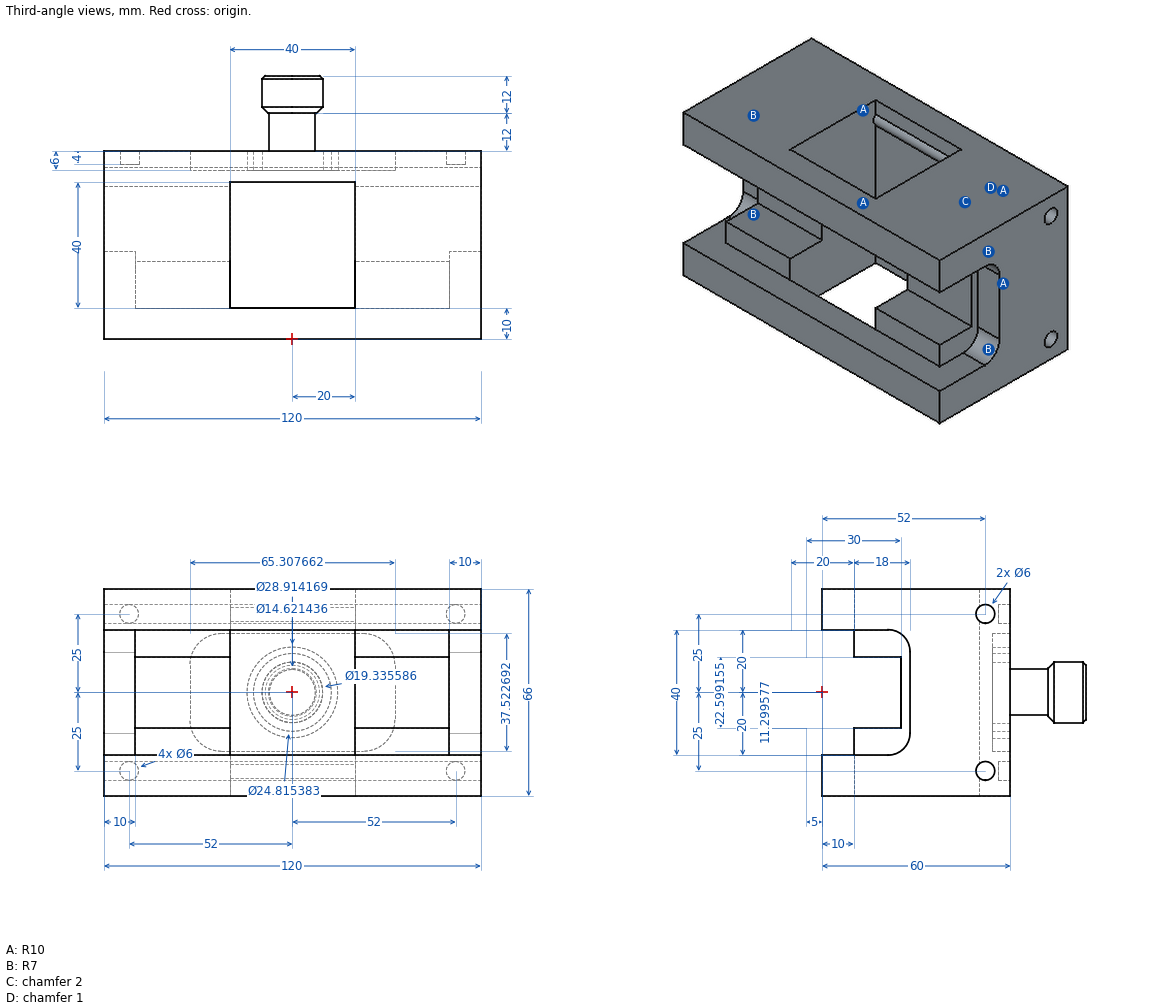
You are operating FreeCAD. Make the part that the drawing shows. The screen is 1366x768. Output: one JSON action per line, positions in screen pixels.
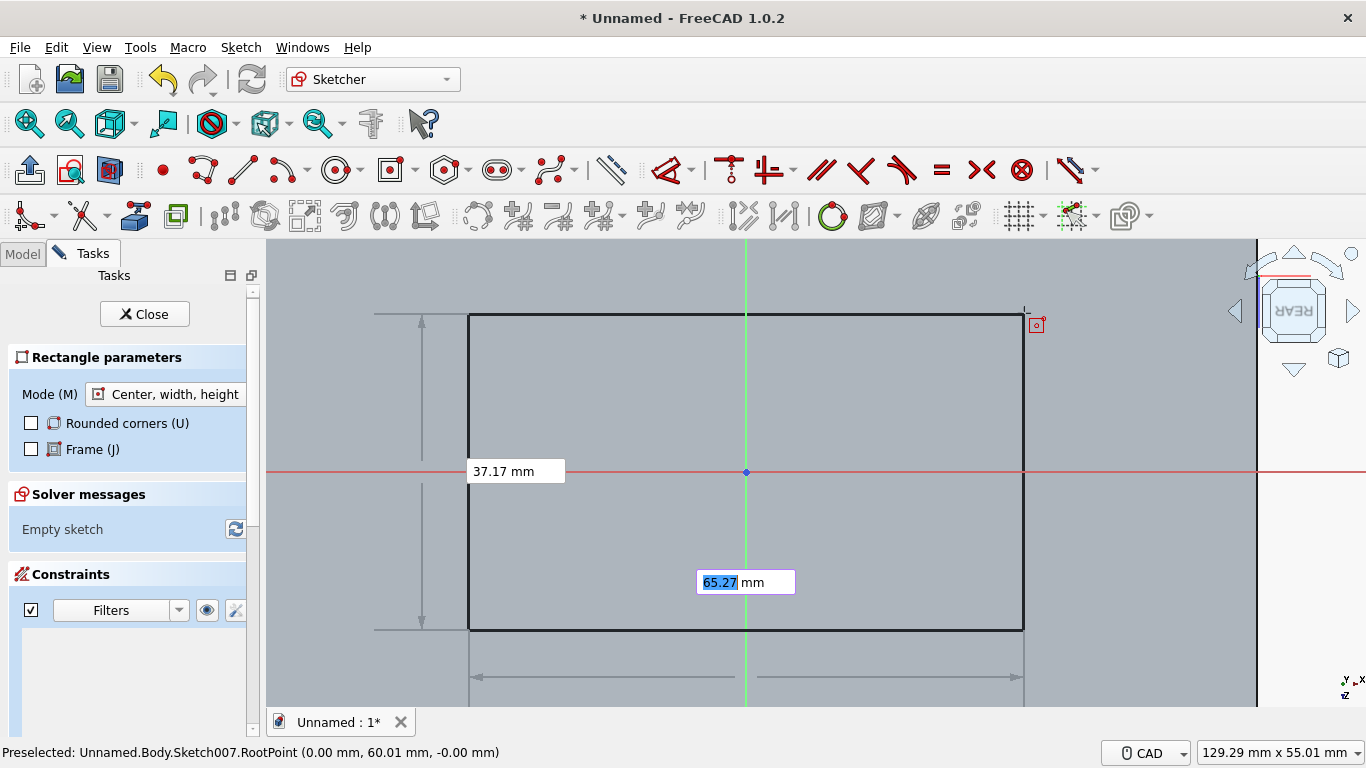
{"action": "type", "text": "65.307662"}
{"action": "key", "text": "Tab"}
{"action": "type", "text": "37.522692"}
{"action": "key", "text": "Return"}
{"action": "key", "text": "Escape"}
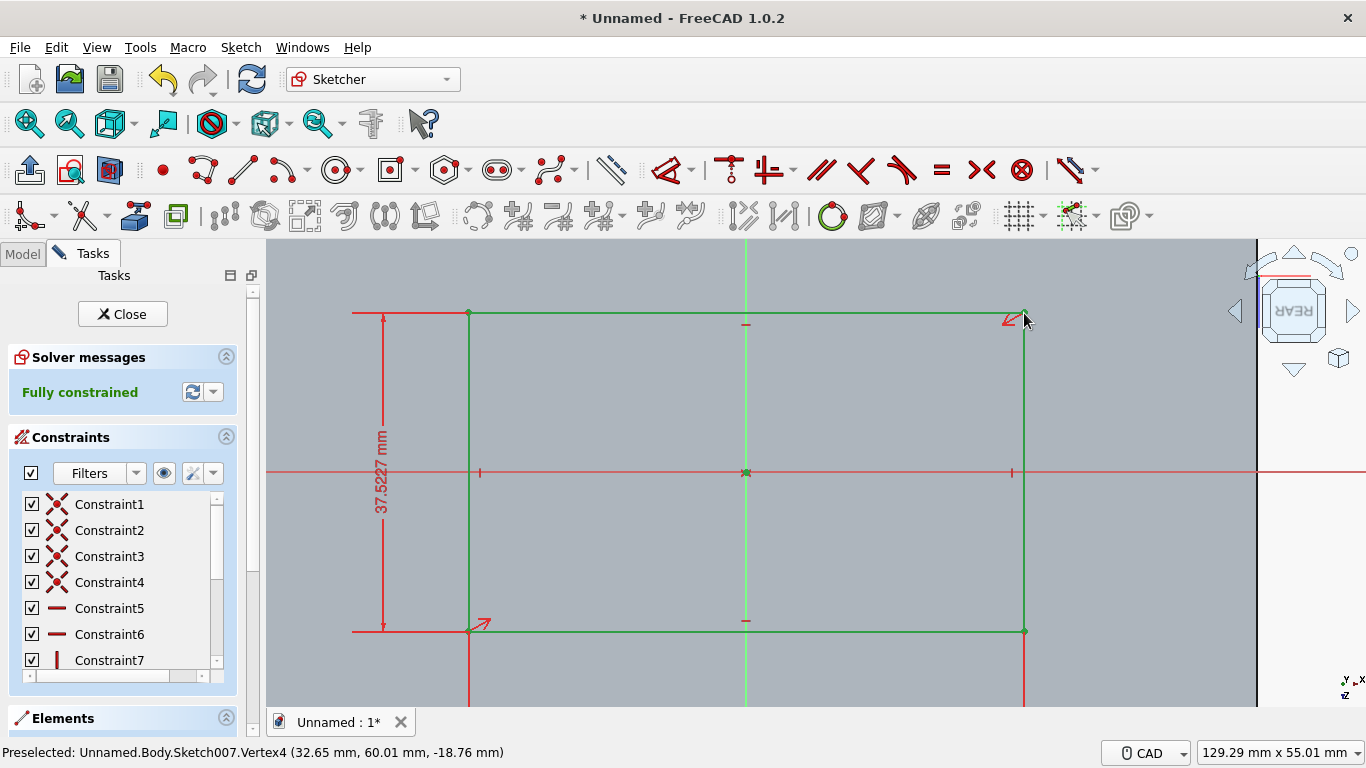
{"action": "left_click", "coordinate": [123, 314]}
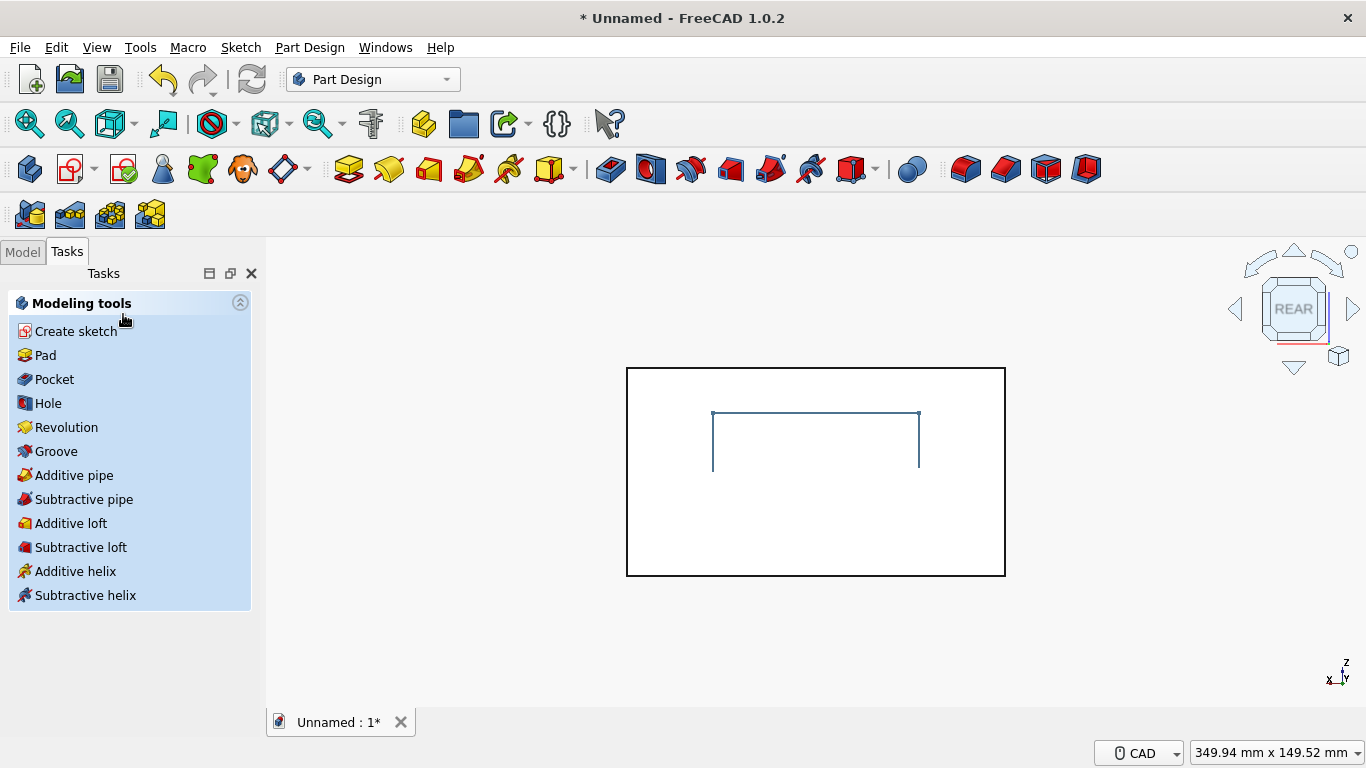
{"action": "left_click", "coordinate": [612, 170]}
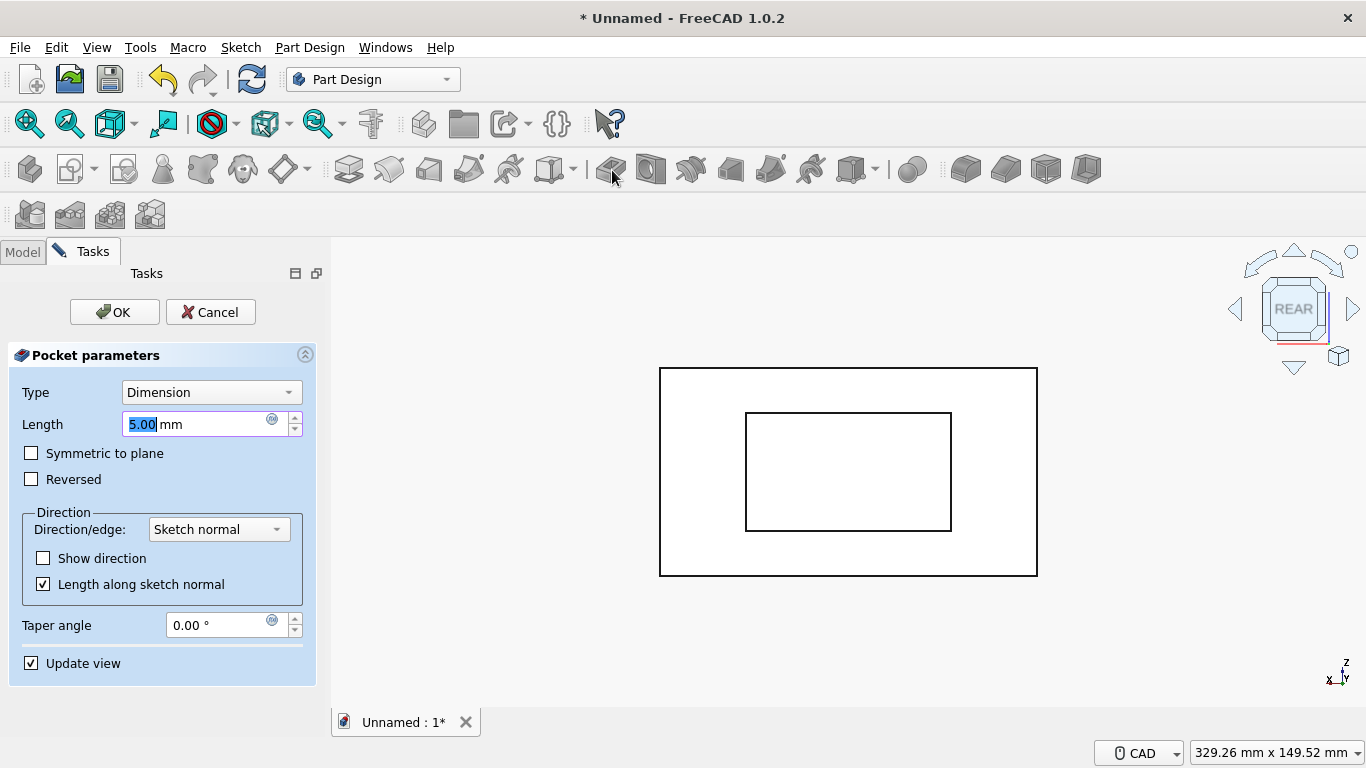
{"action": "type", "text": "6"}
{"action": "key", "text": "Tab"}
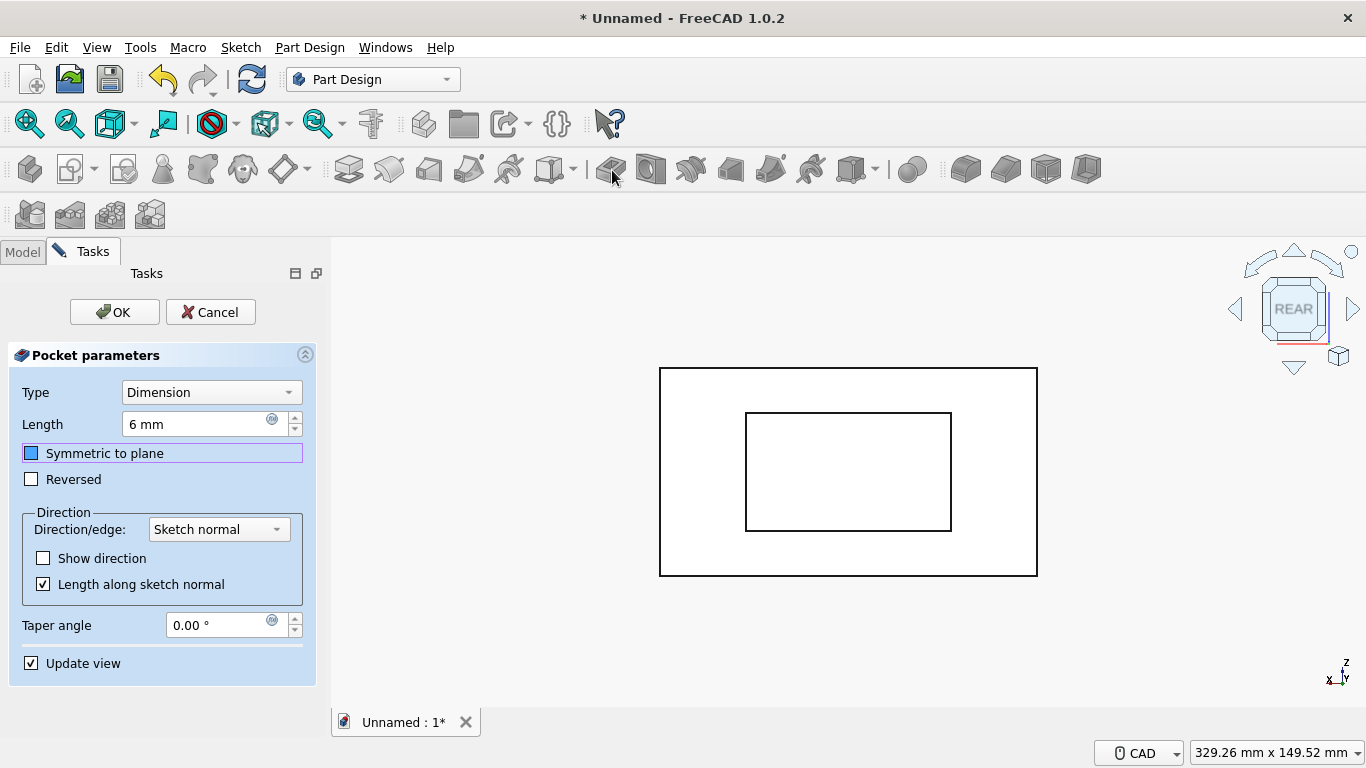
{"action": "left_click", "coordinate": [115, 312]}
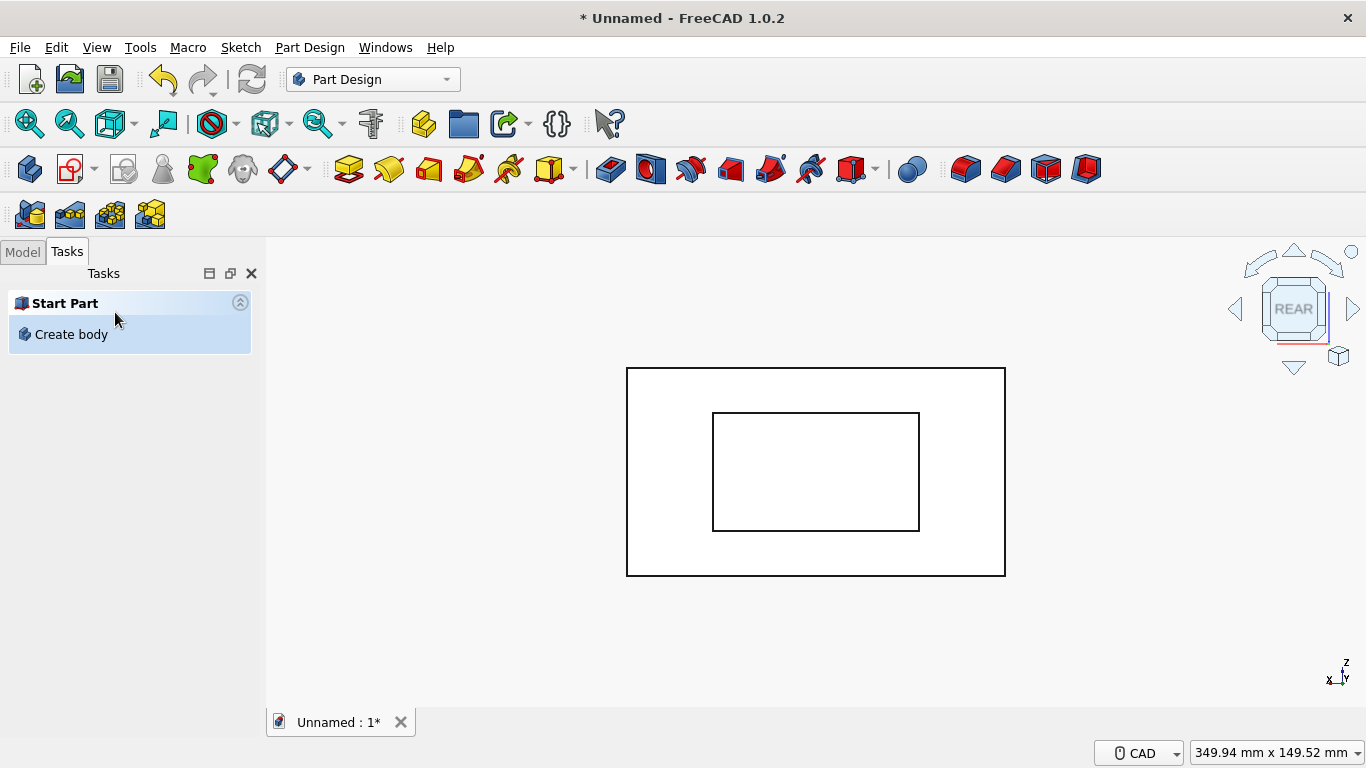
{"action": "left_click", "coordinate": [30, 124]}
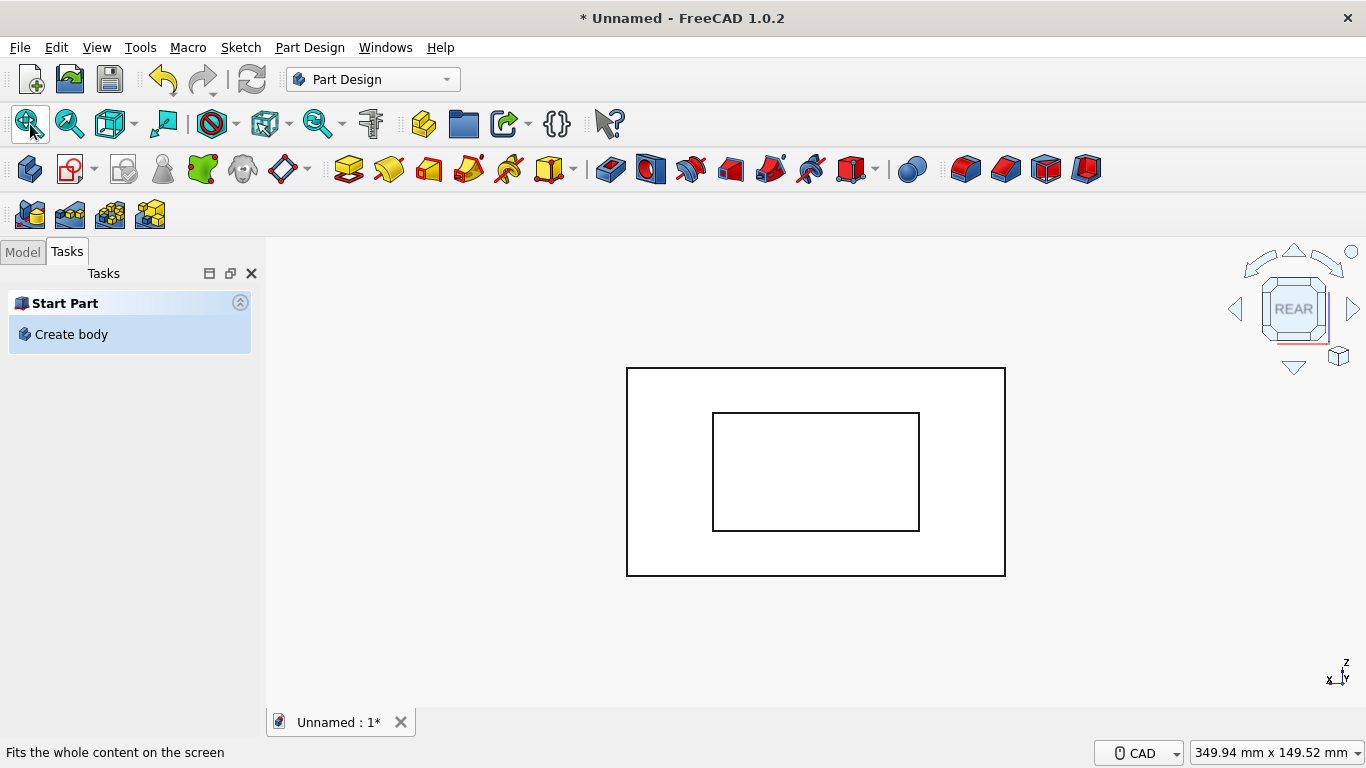
{"action": "scroll", "coordinate": [713, 530], "scroll_direction": "up", "scroll_amount": 4}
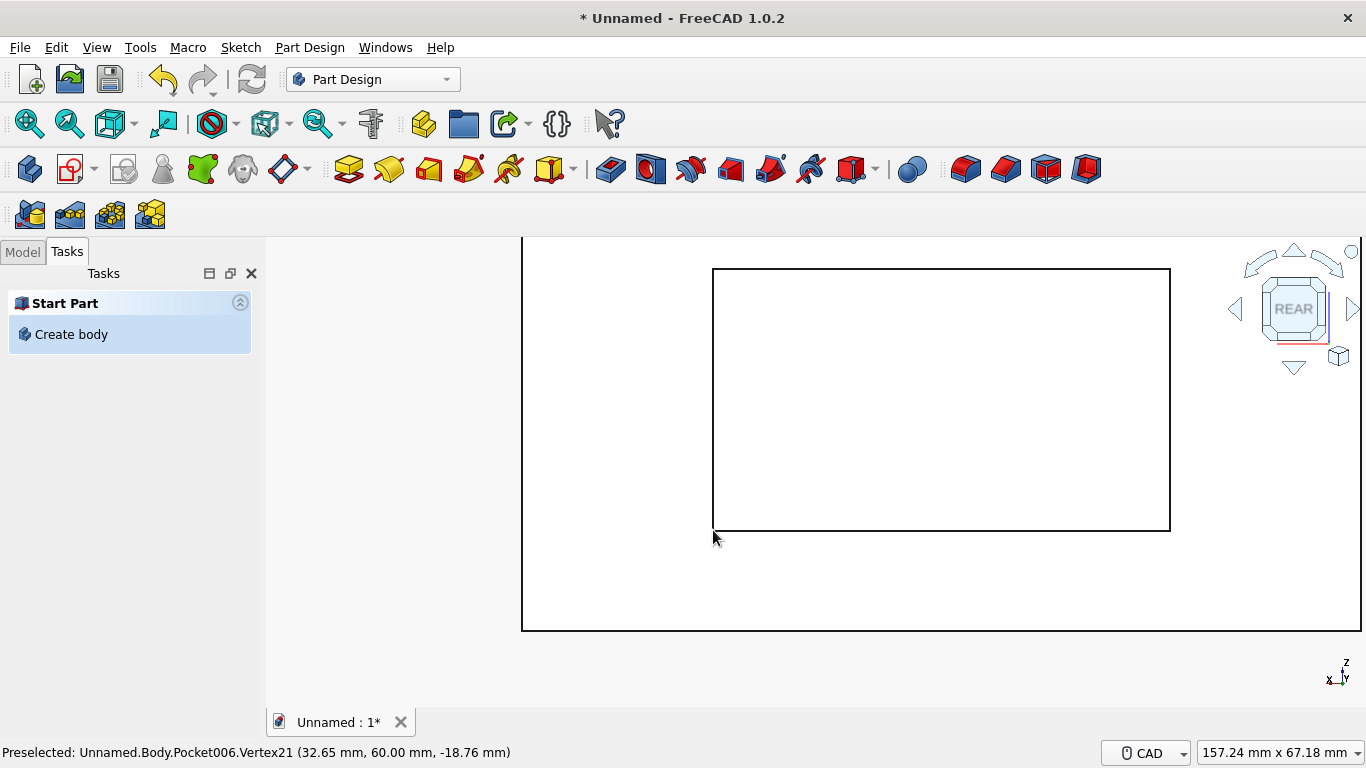
{"action": "left_click", "coordinate": [30, 124]}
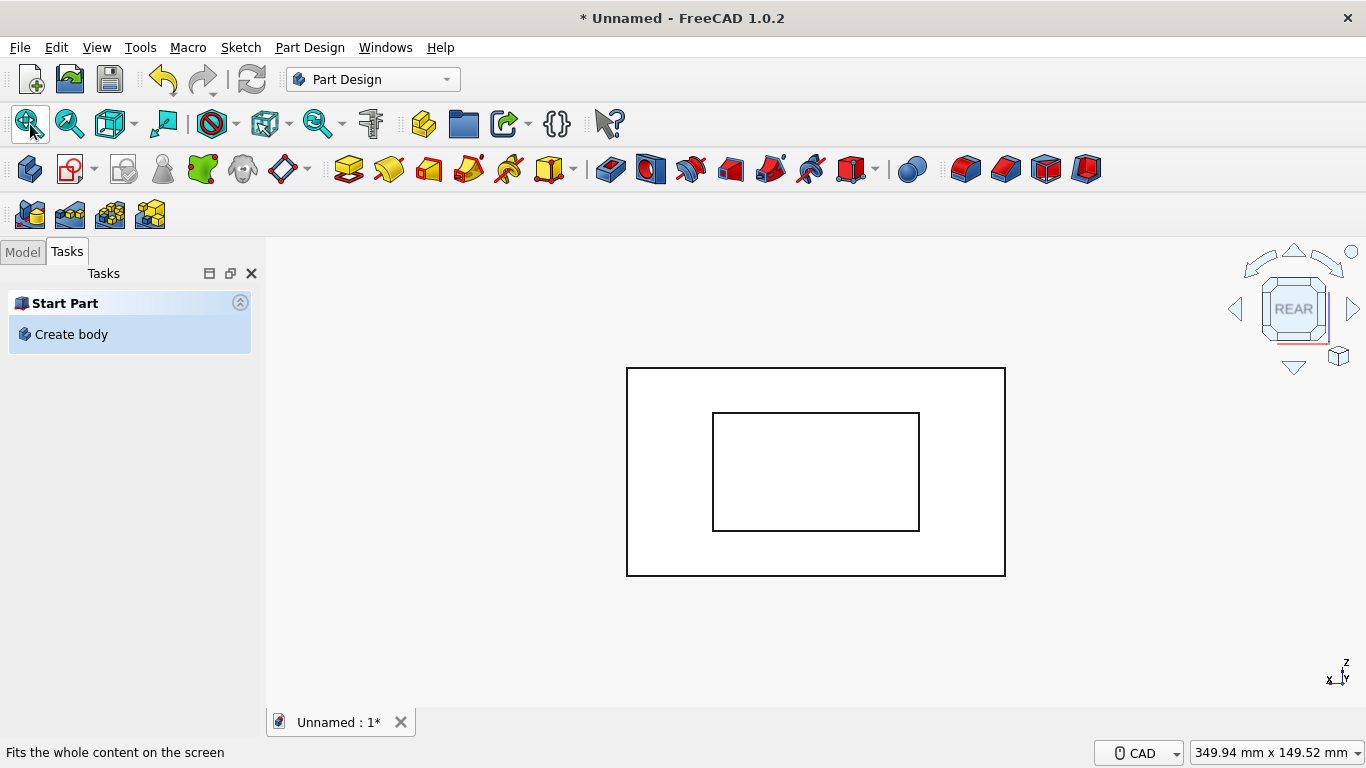
{"action": "key", "text": "0"}